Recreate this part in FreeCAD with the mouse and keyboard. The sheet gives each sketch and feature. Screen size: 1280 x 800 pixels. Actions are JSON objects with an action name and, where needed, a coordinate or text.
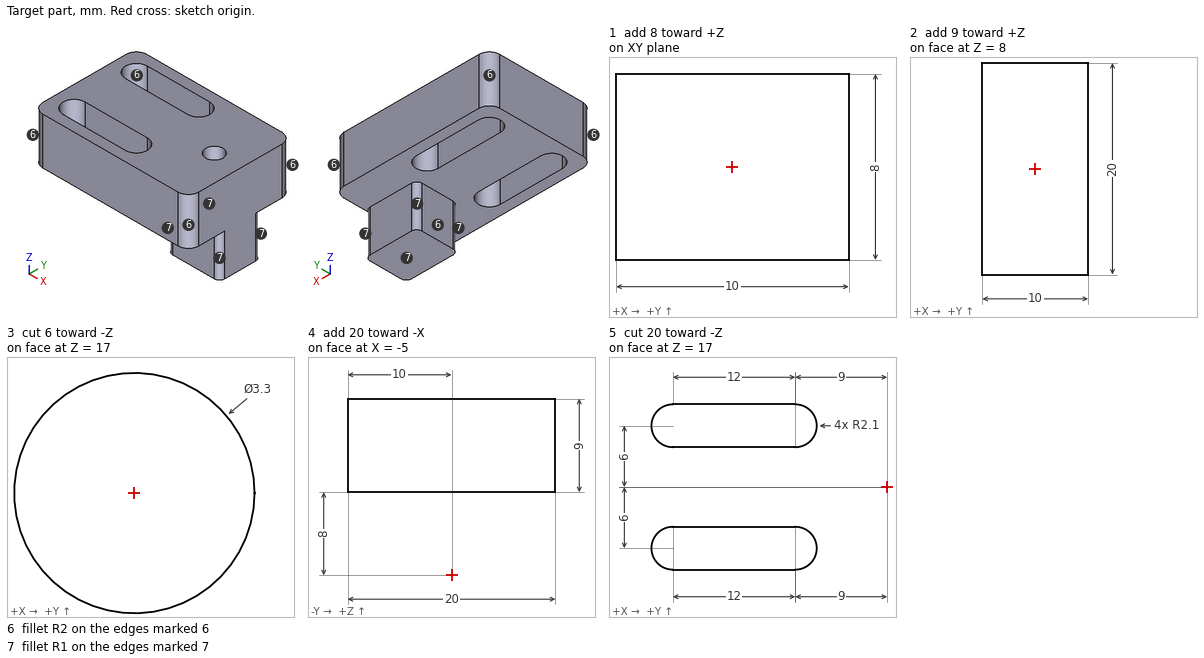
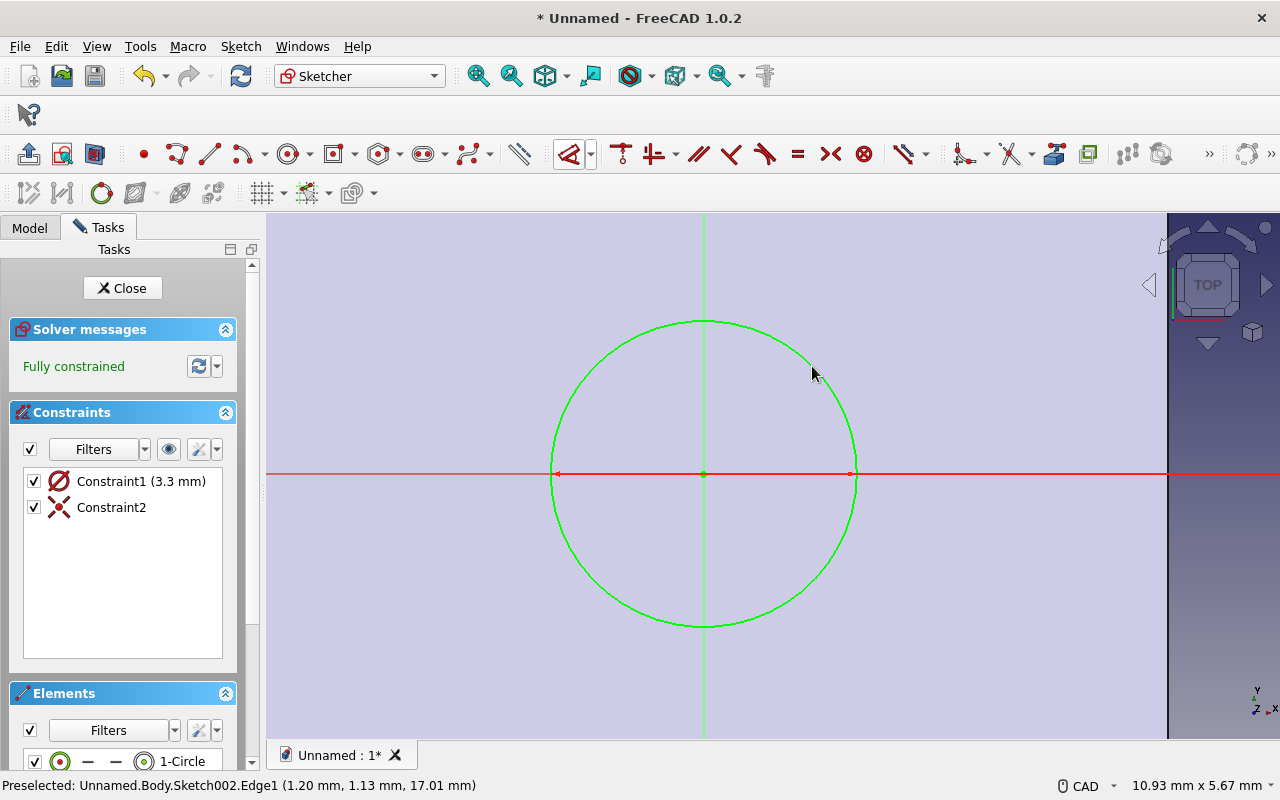
{"action": "left_click", "coordinate": [123, 288]}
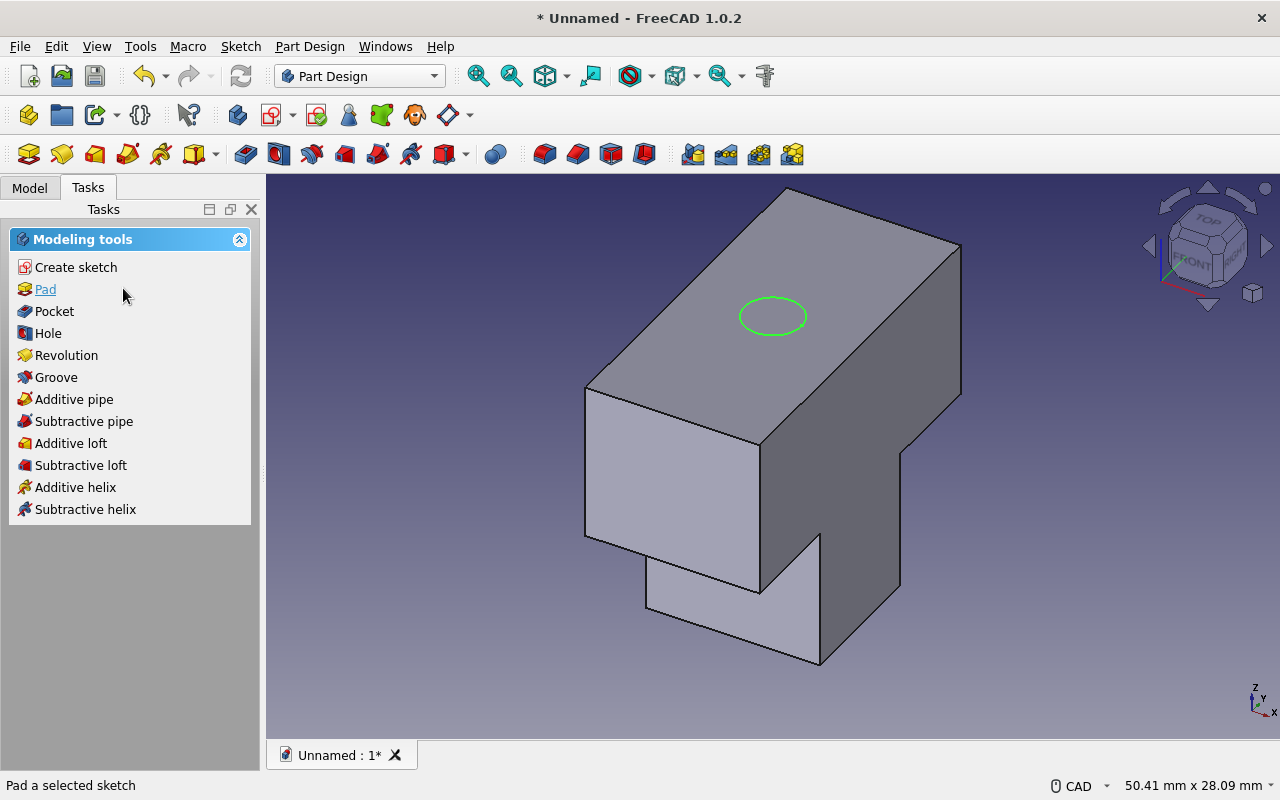
{"action": "left_click", "coordinate": [246, 154]}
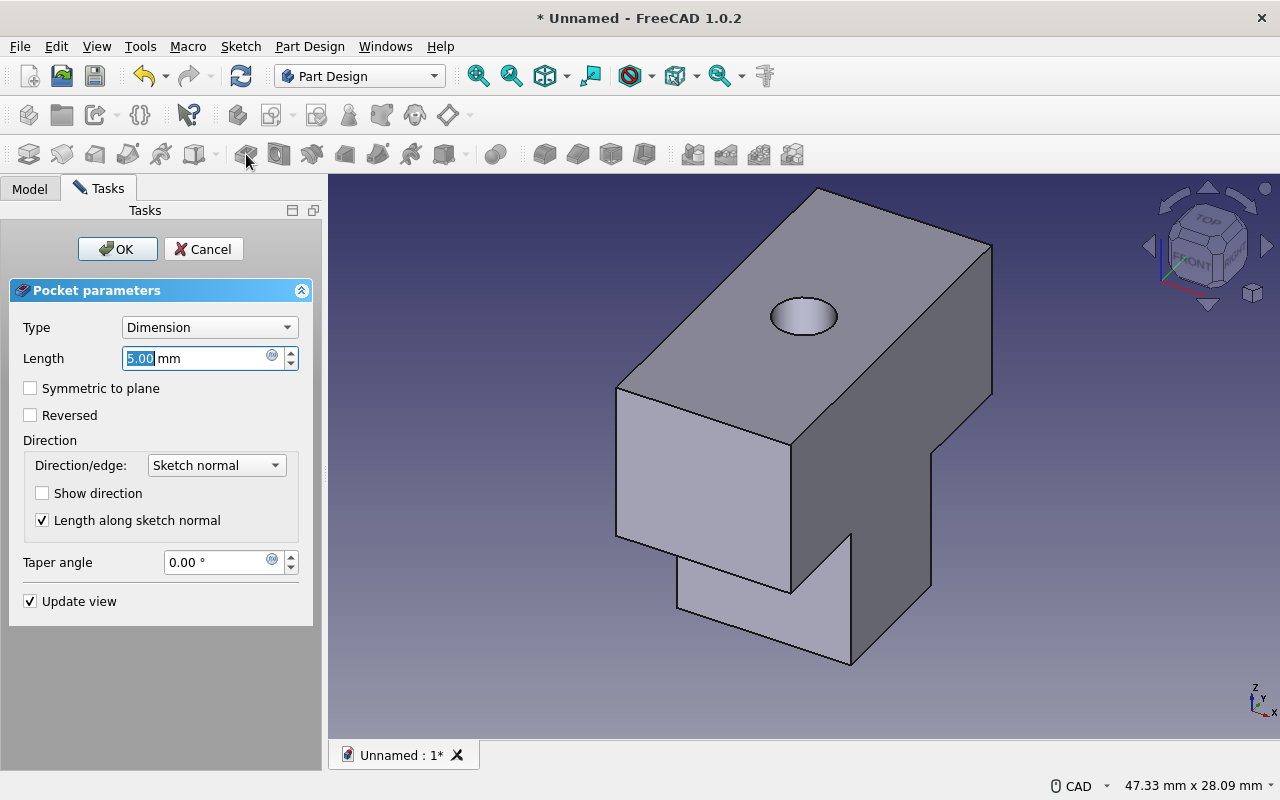
{"action": "type", "text": "6"}
{"action": "key", "text": "Tab"}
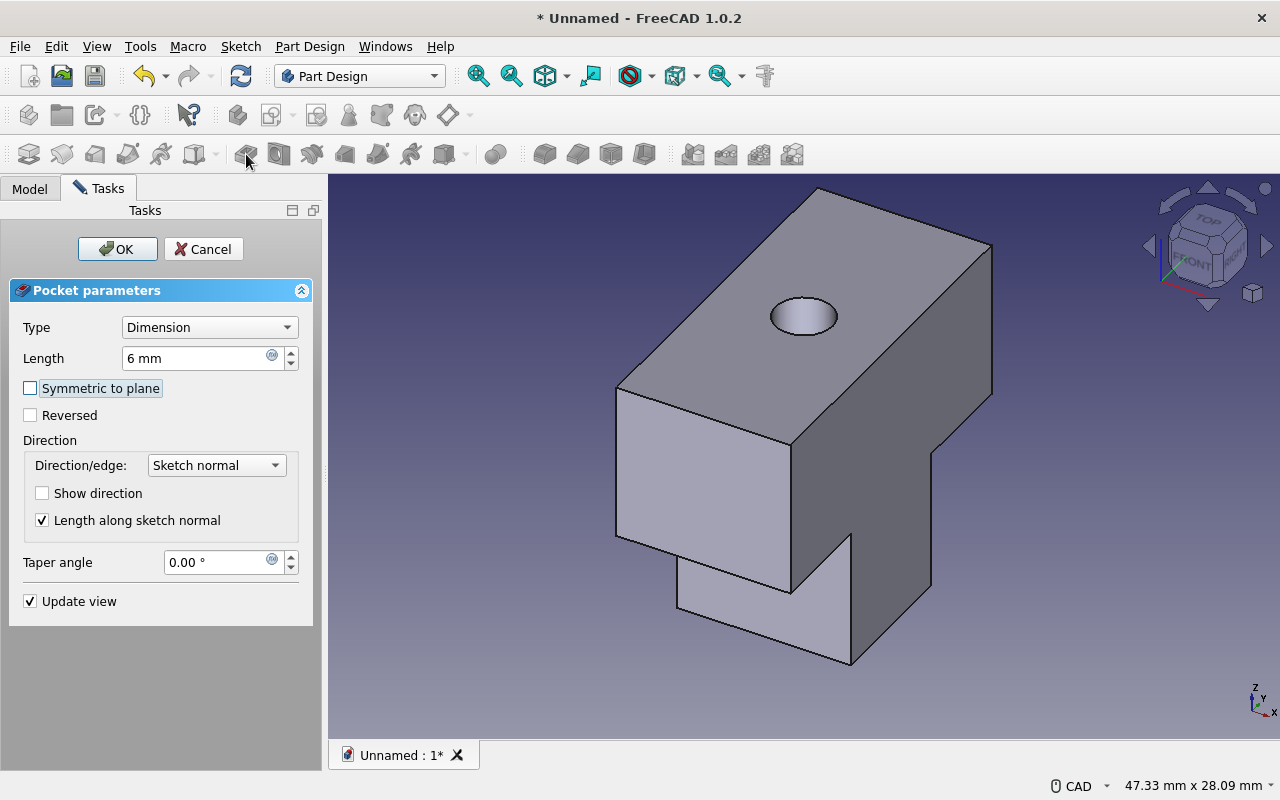
{"action": "left_click", "coordinate": [118, 249]}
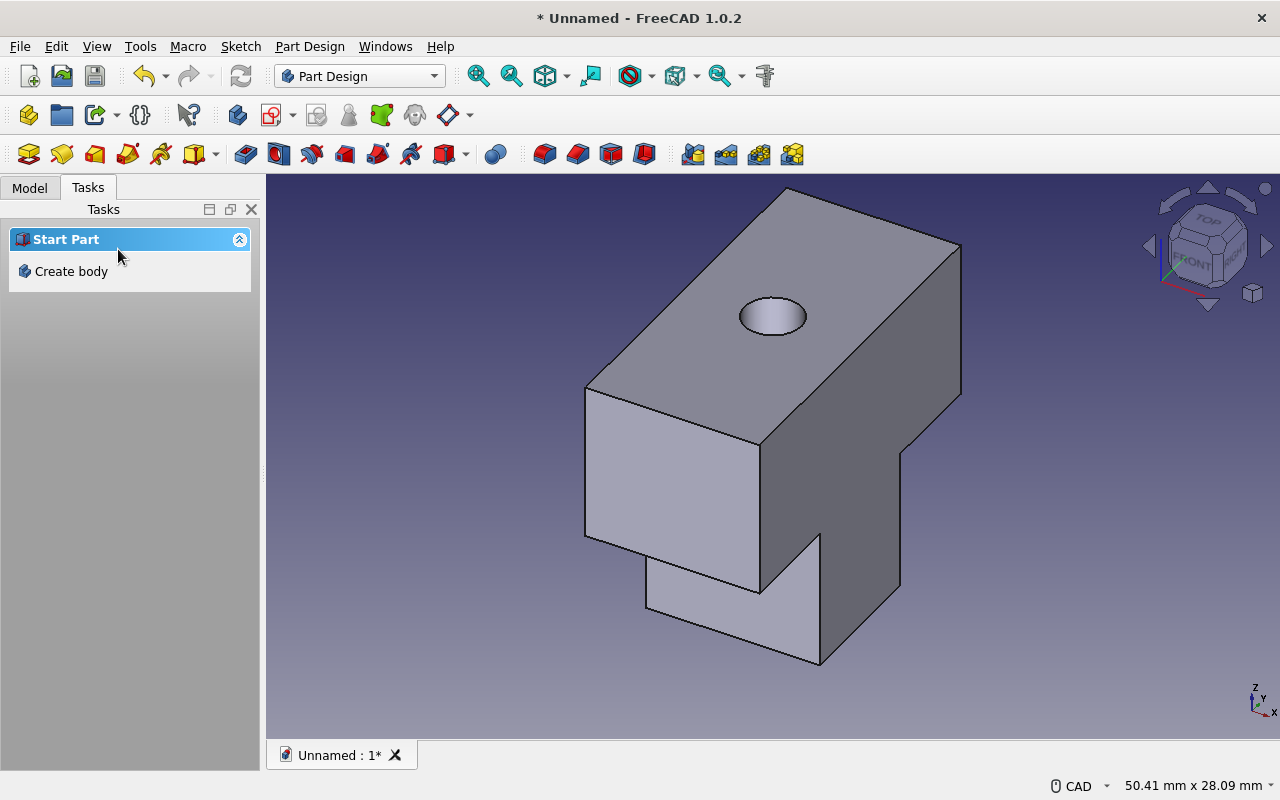
{"action": "key", "text": "6"}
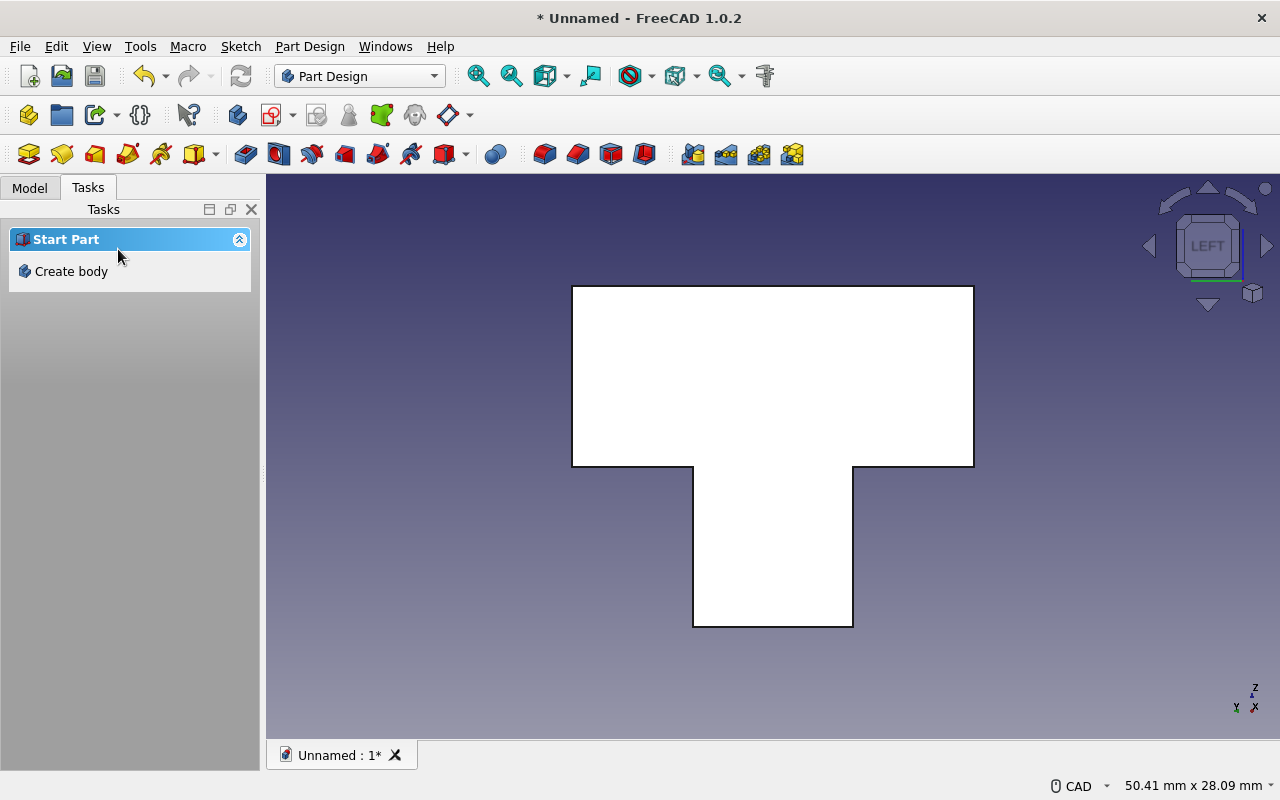
{"action": "left_click", "coordinate": [773, 407]}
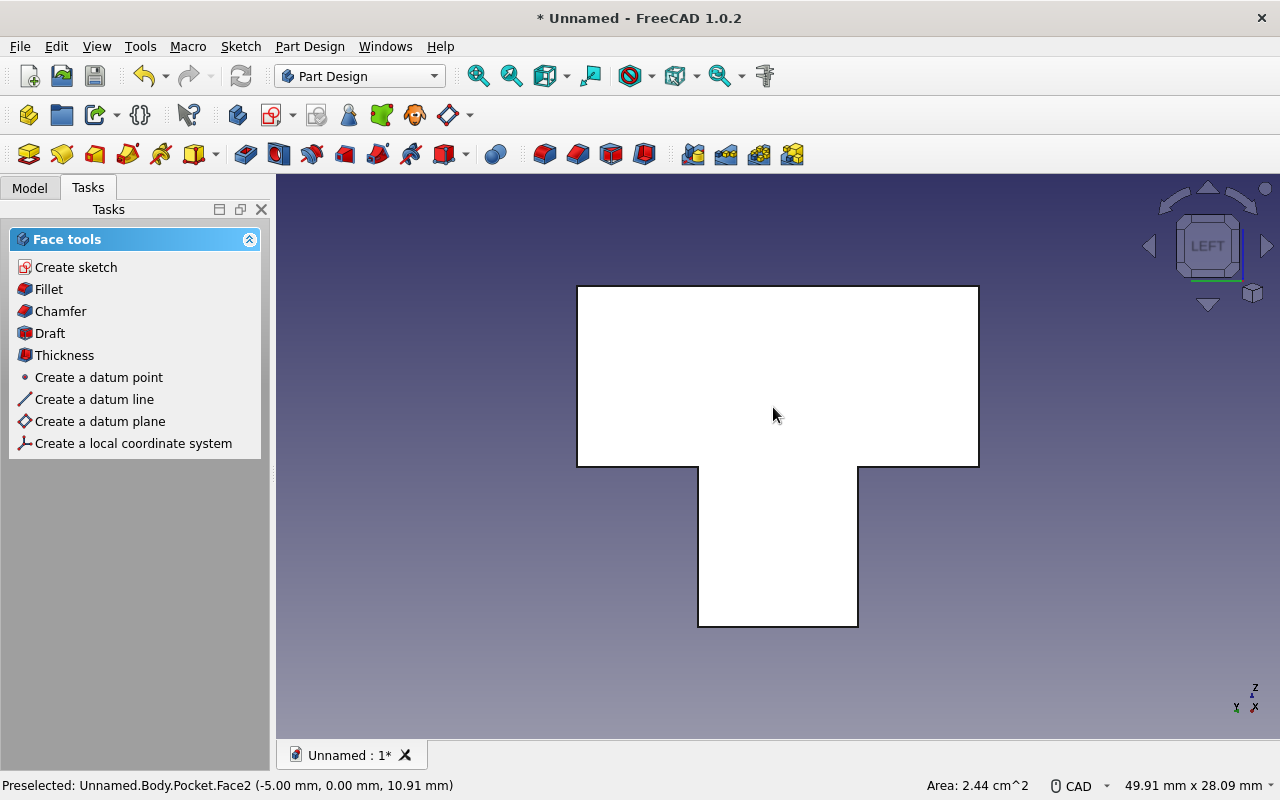
{"action": "left_click", "coordinate": [270, 116]}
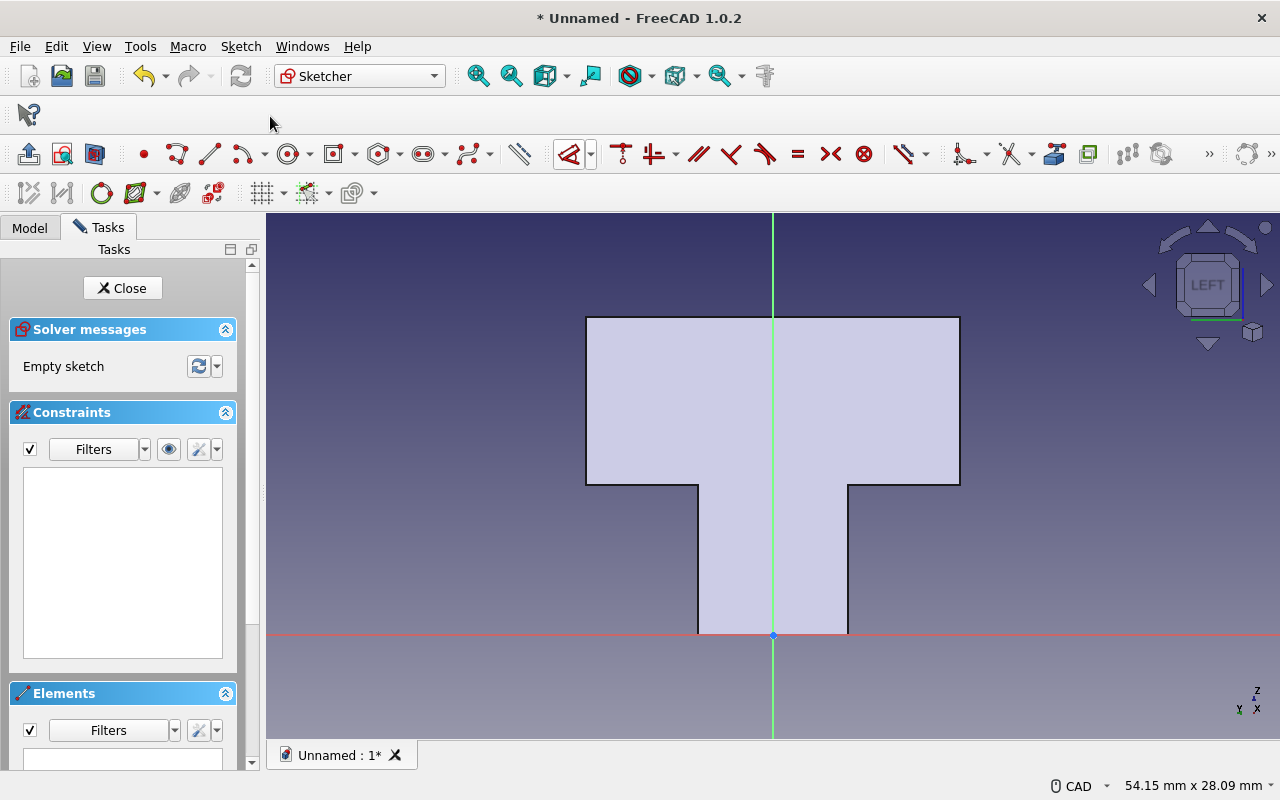
{"action": "left_click", "coordinate": [354, 154]}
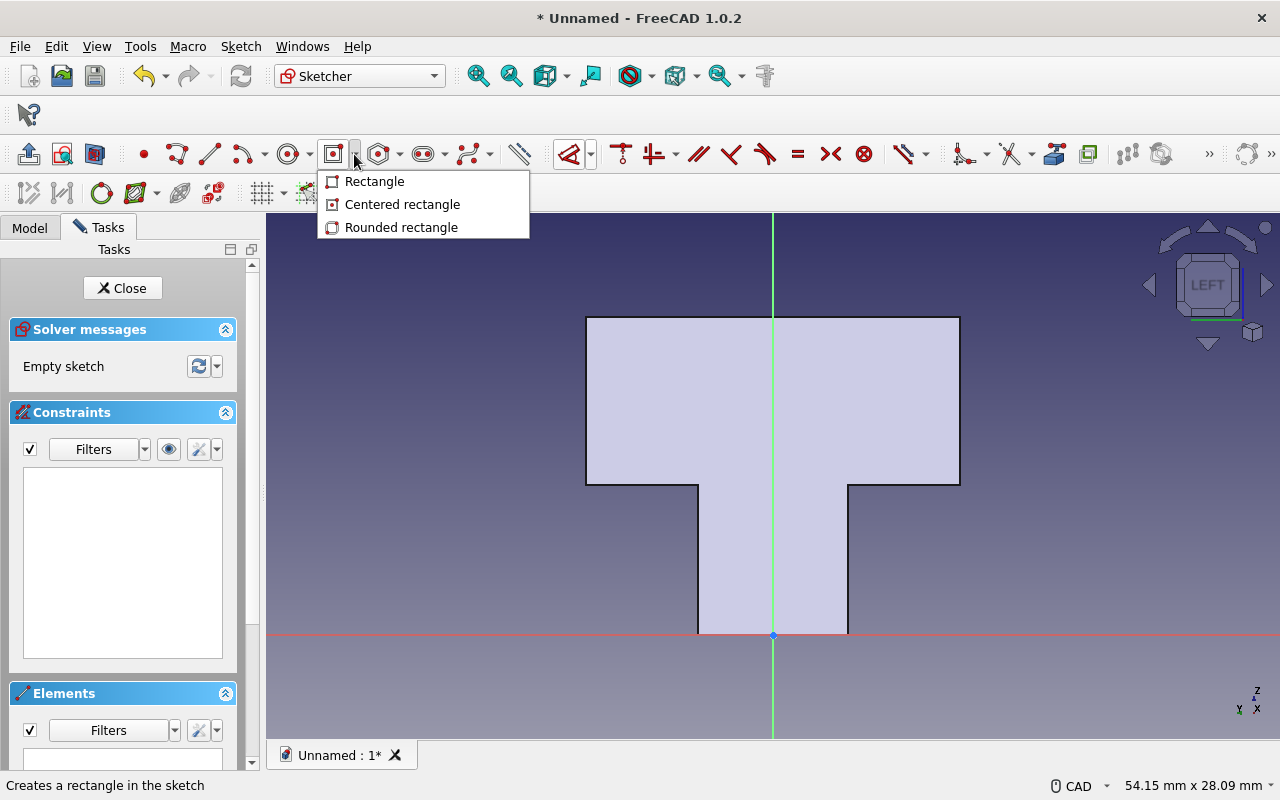
{"action": "left_click", "coordinate": [424, 182]}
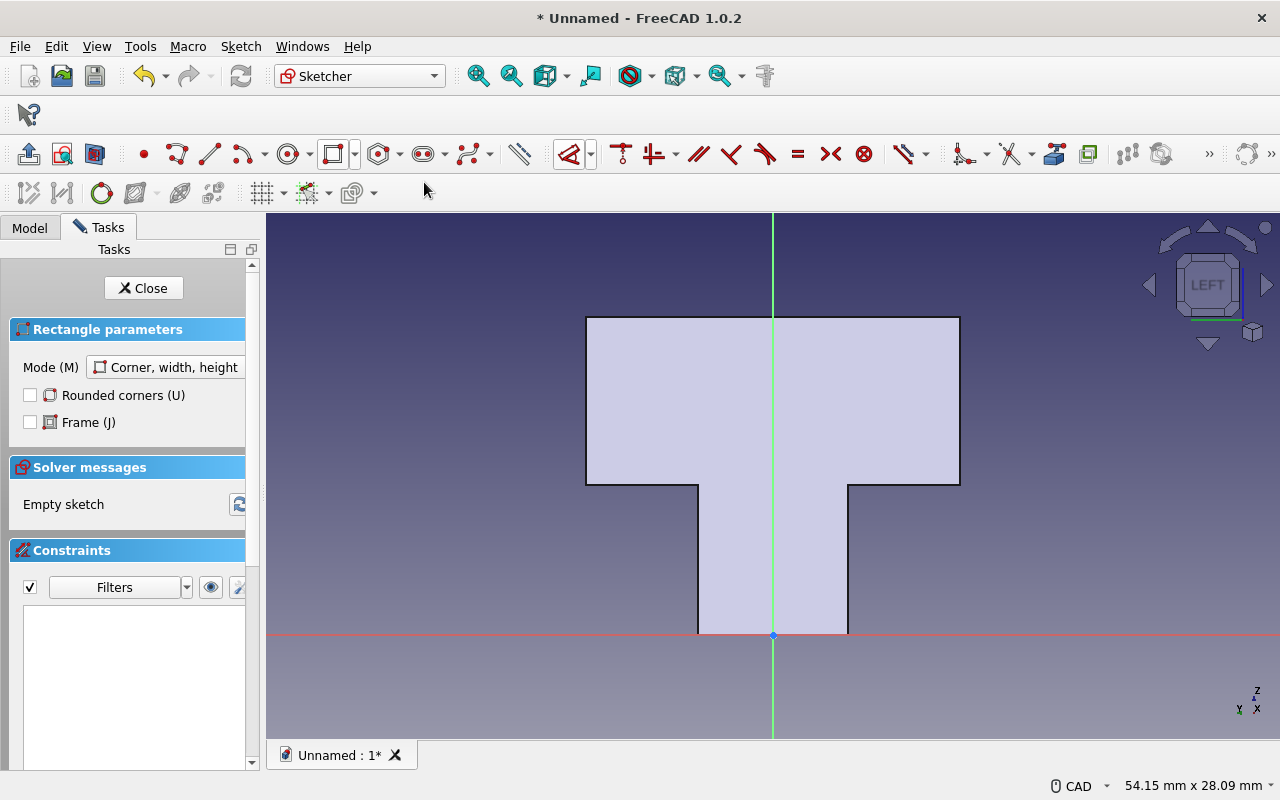
{"action": "left_click", "coordinate": [586, 317]}
{"action": "mouse_move", "coordinate": [960, 485]}